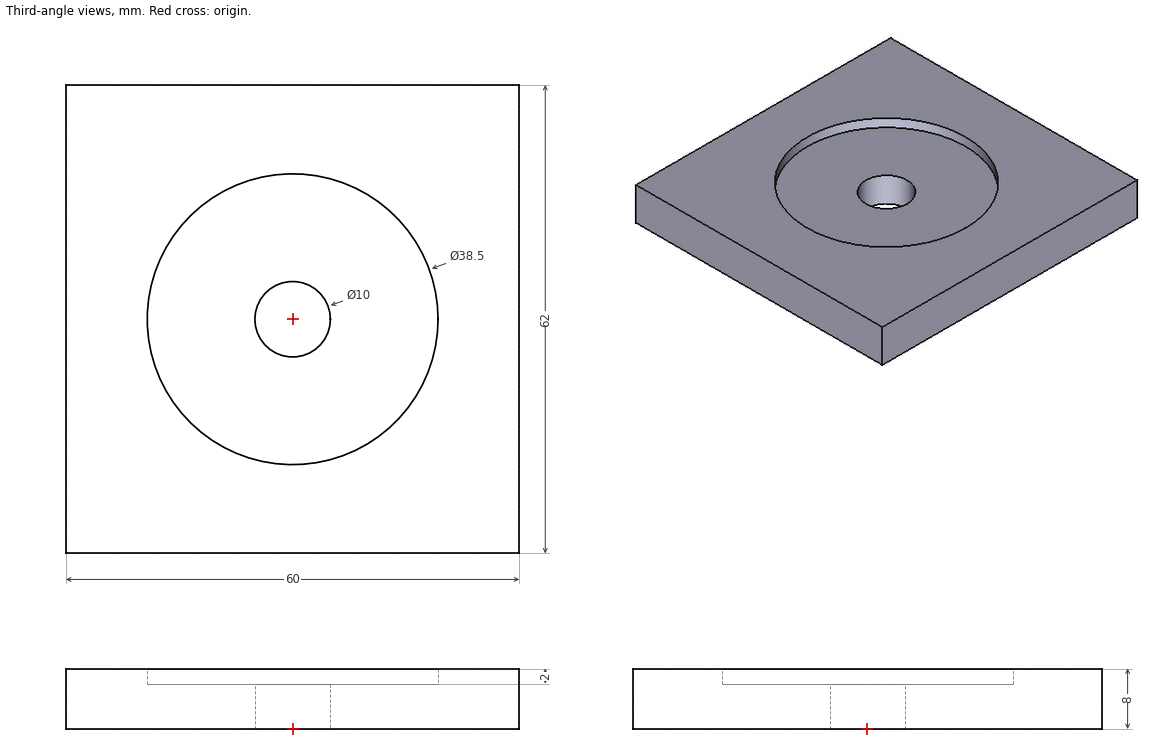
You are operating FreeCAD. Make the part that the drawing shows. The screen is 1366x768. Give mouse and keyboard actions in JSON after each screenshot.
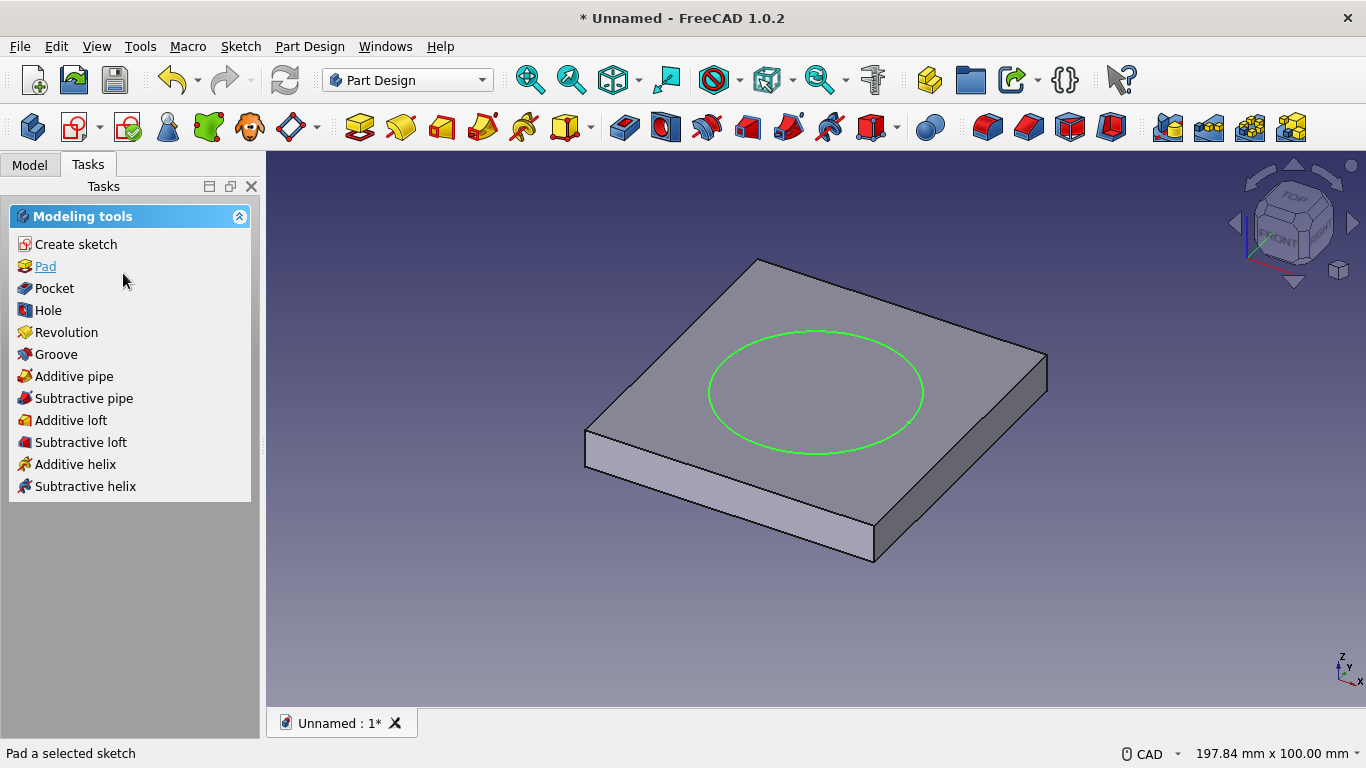
{"action": "left_click", "coordinate": [625, 128]}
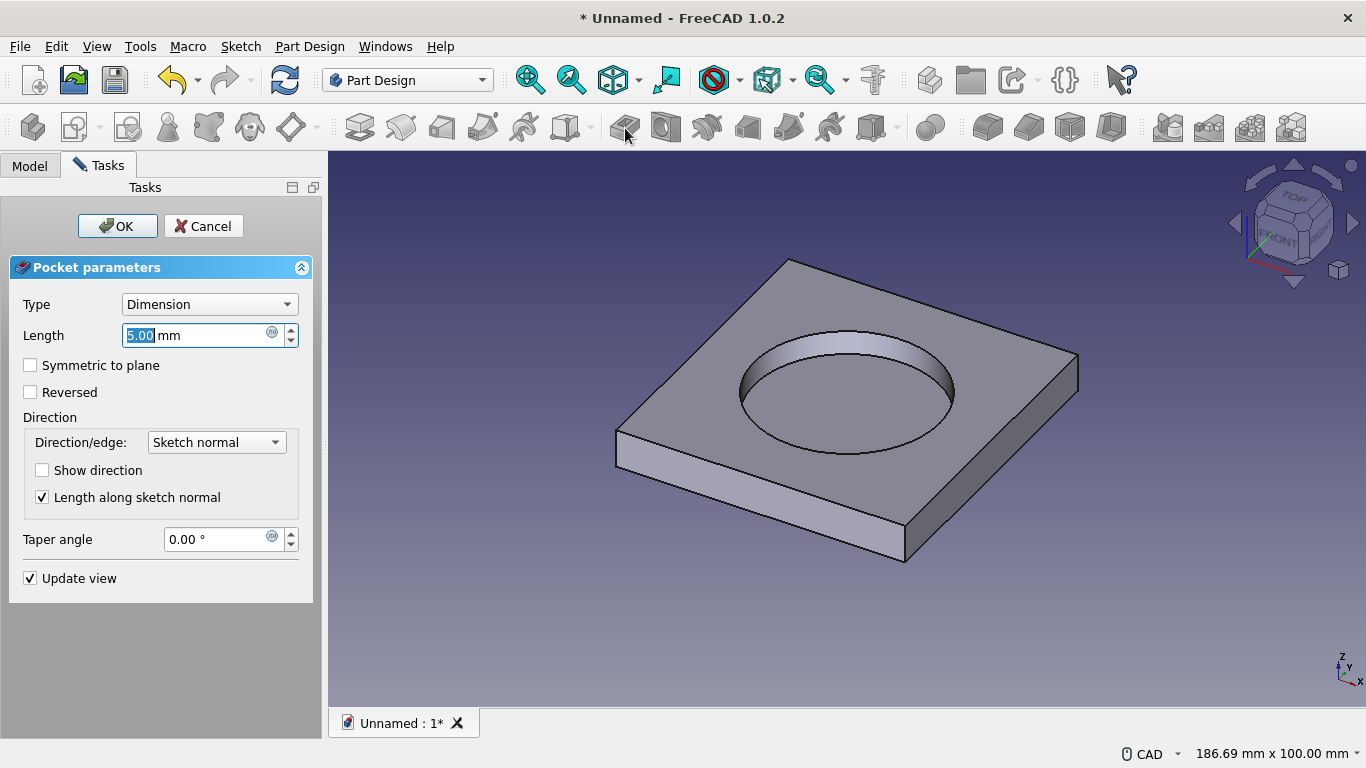
{"action": "type", "text": "2"}
{"action": "key", "text": "Tab"}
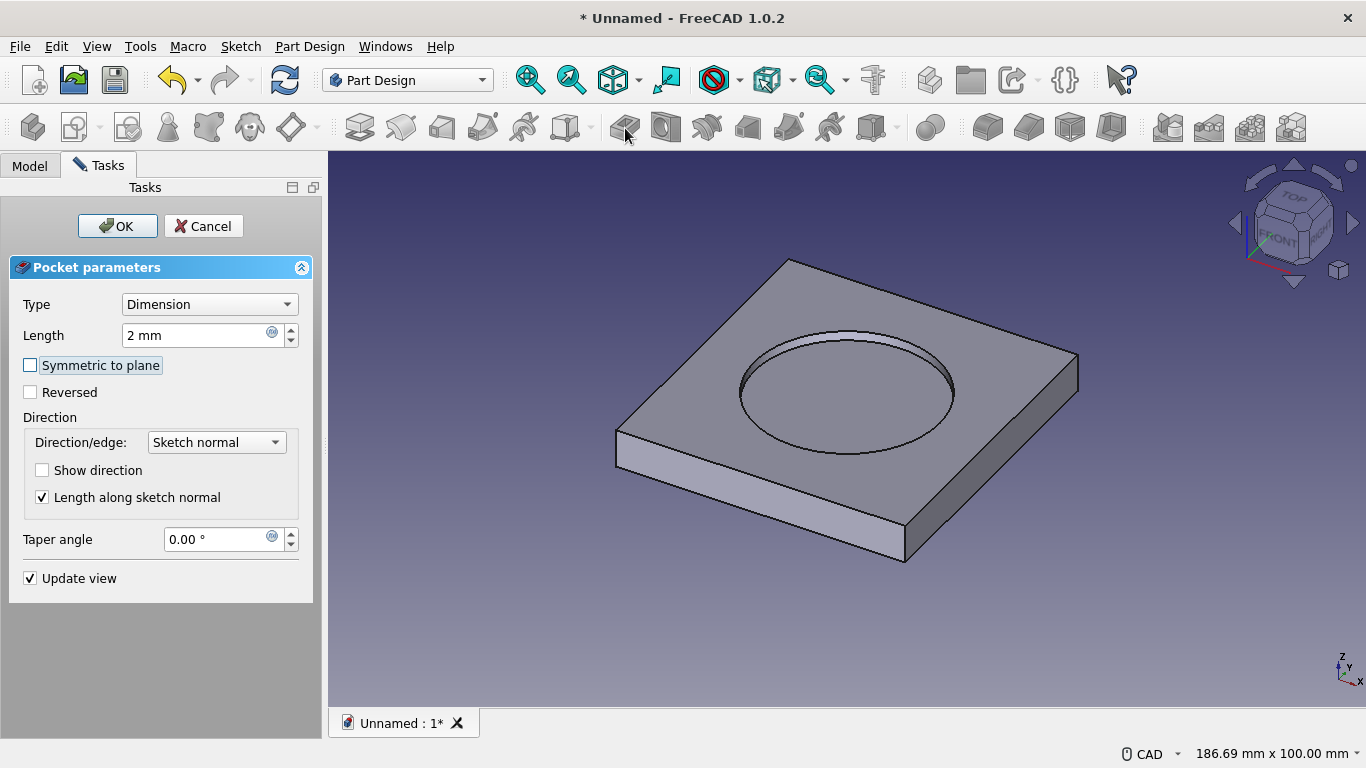
{"action": "left_click", "coordinate": [118, 226]}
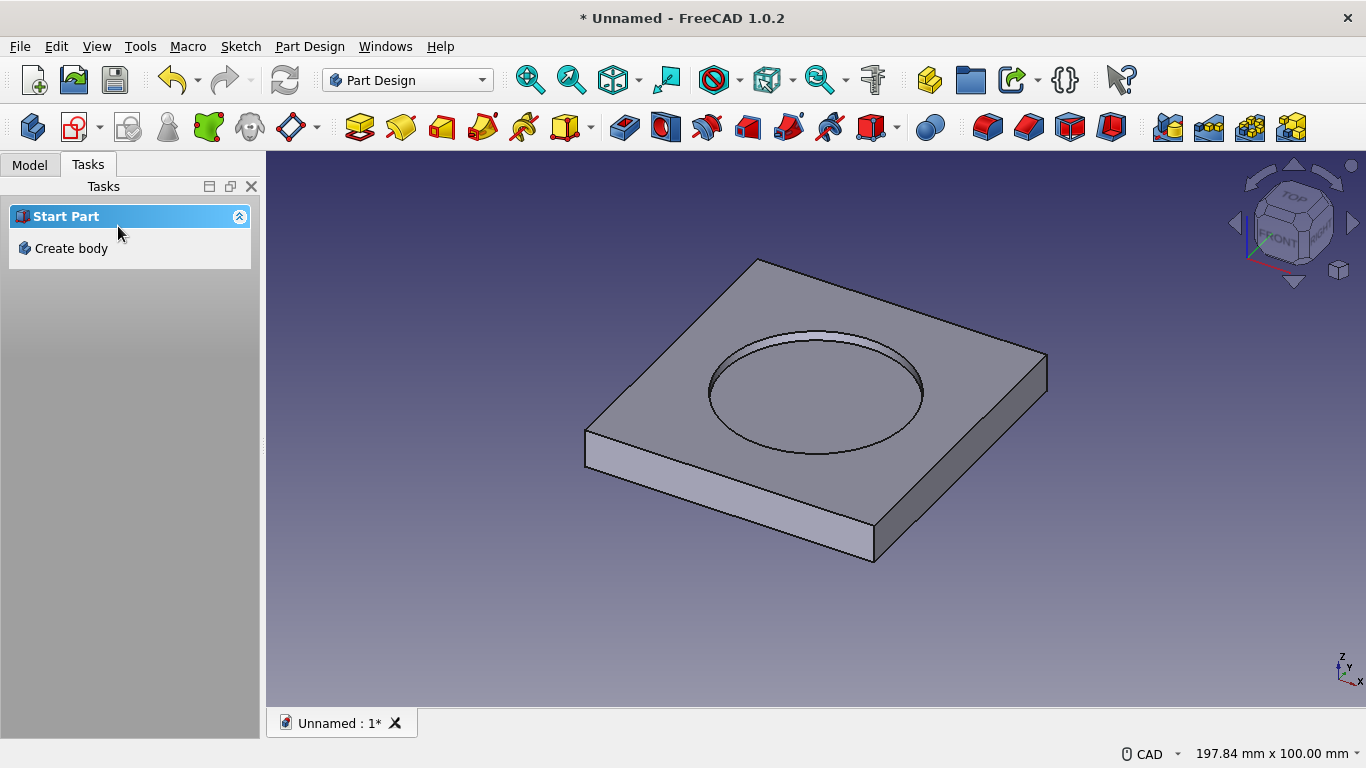
{"action": "left_click", "coordinate": [816, 401]}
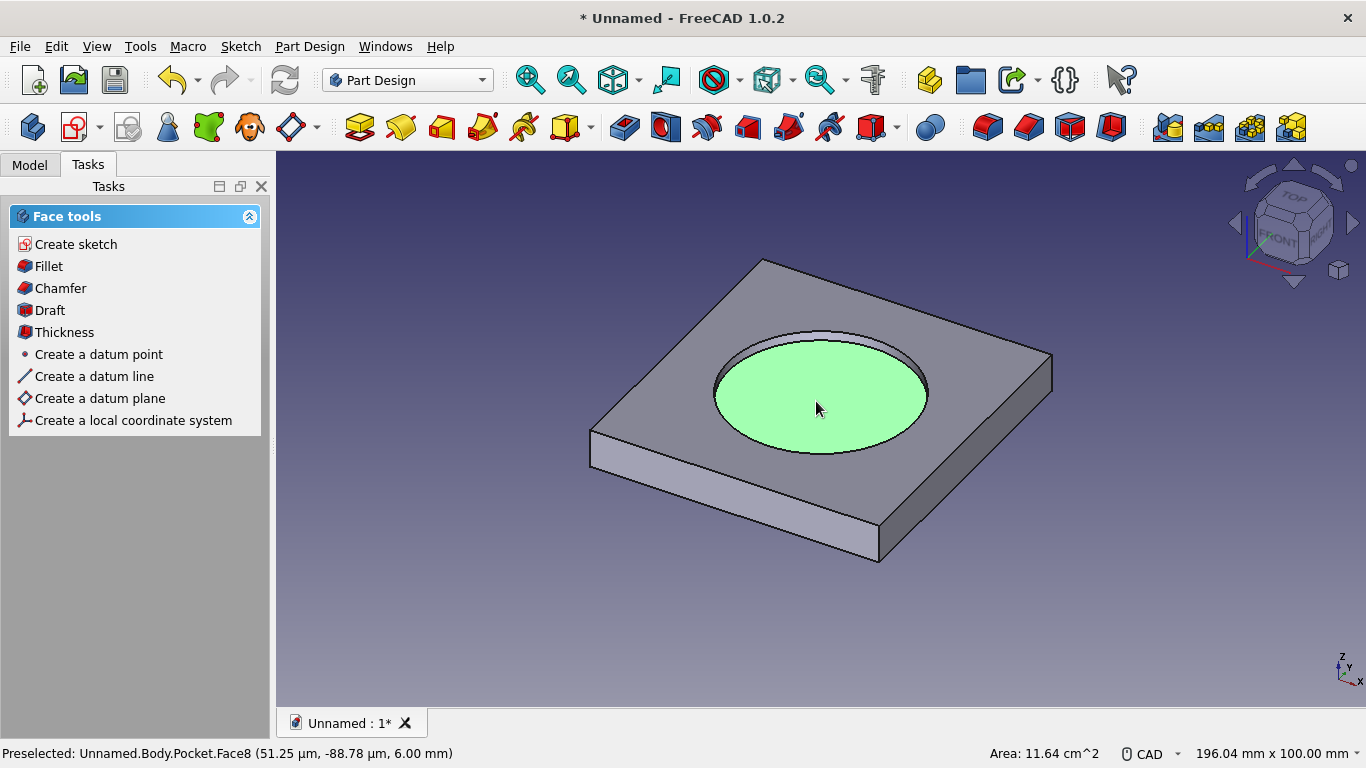
{"action": "left_click", "coordinate": [74, 128]}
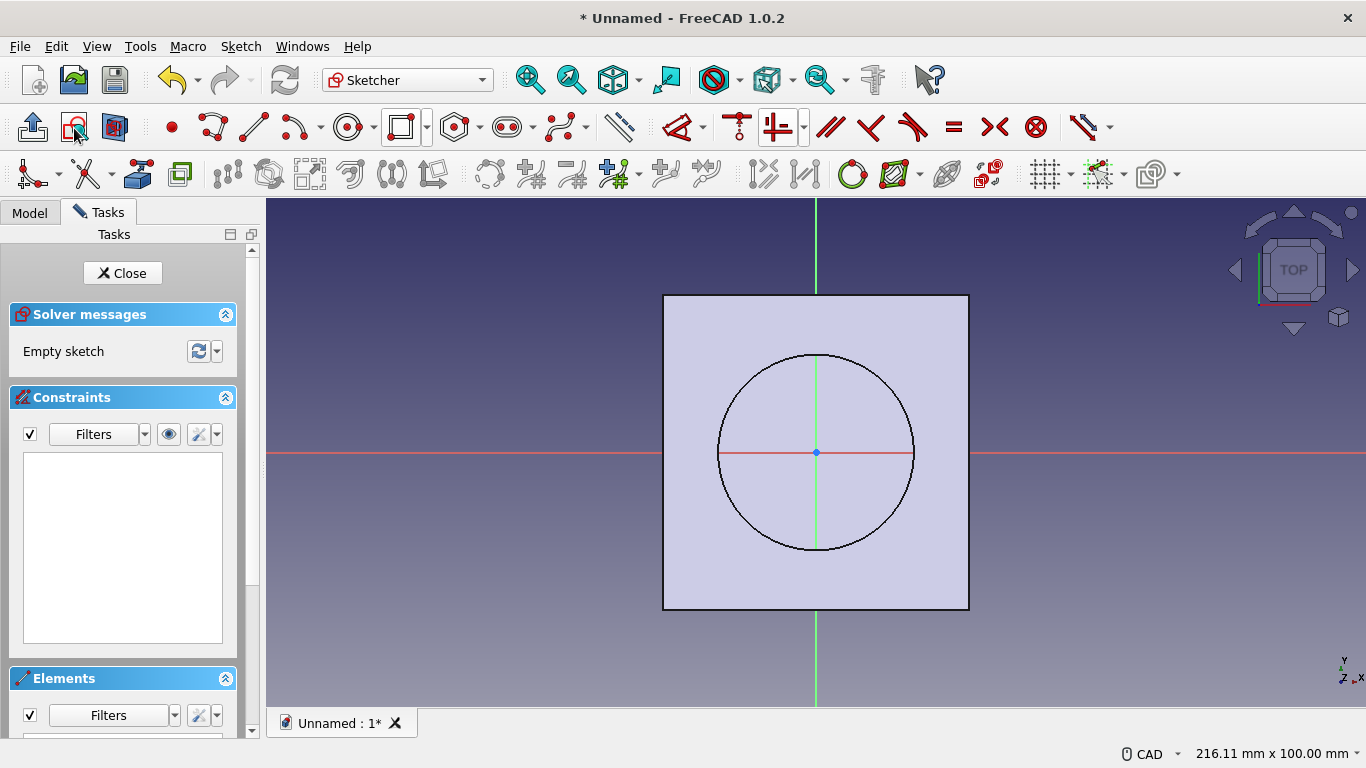
{"action": "left_click", "coordinate": [115, 128]}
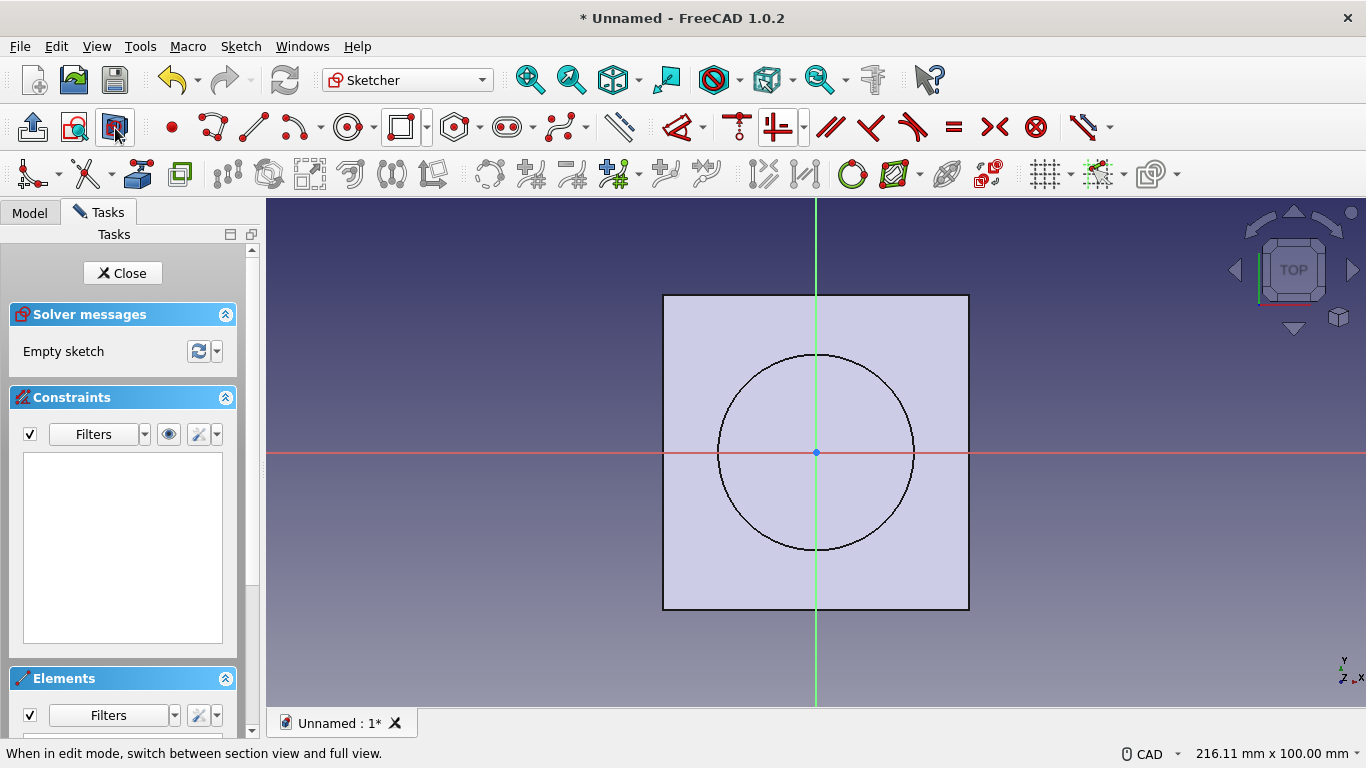
{"action": "scroll", "coordinate": [830, 452], "scroll_direction": "up", "scroll_amount": 9}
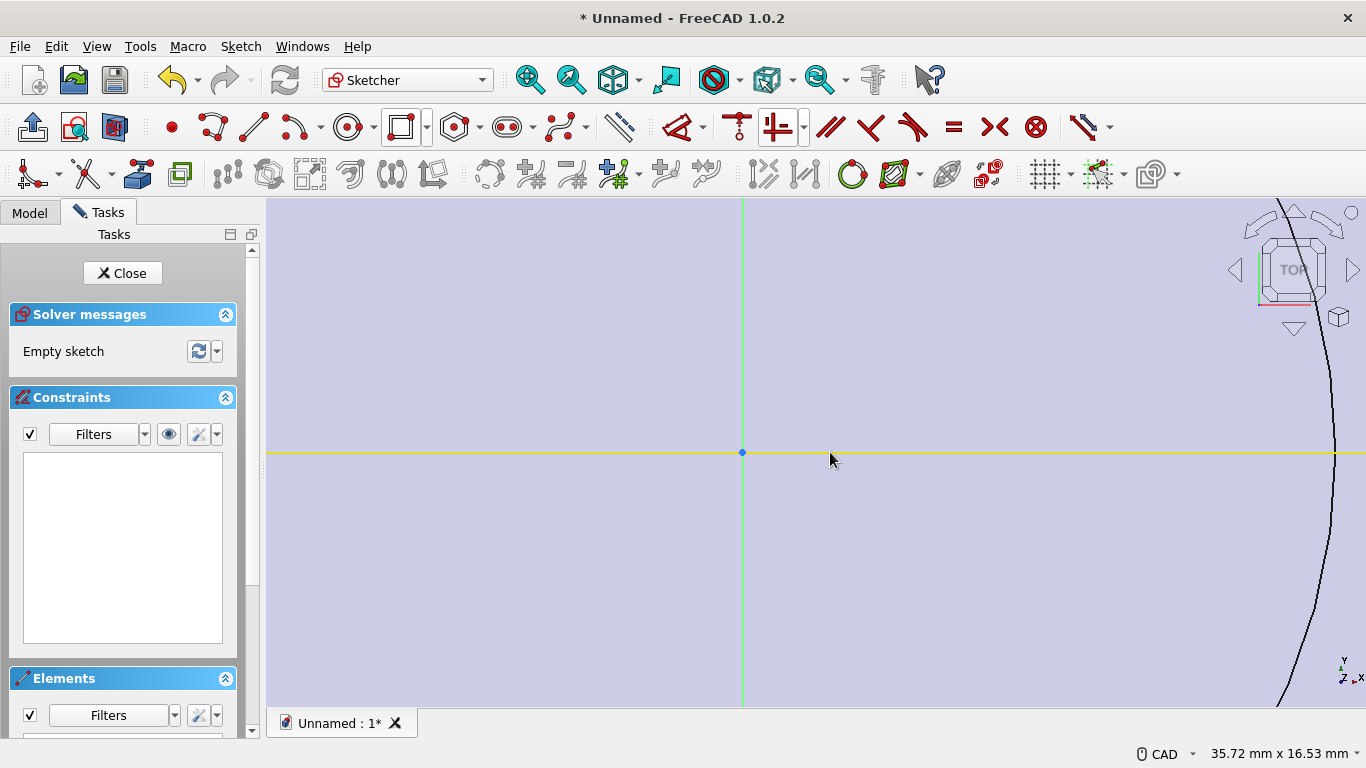
{"action": "left_click", "coordinate": [348, 128]}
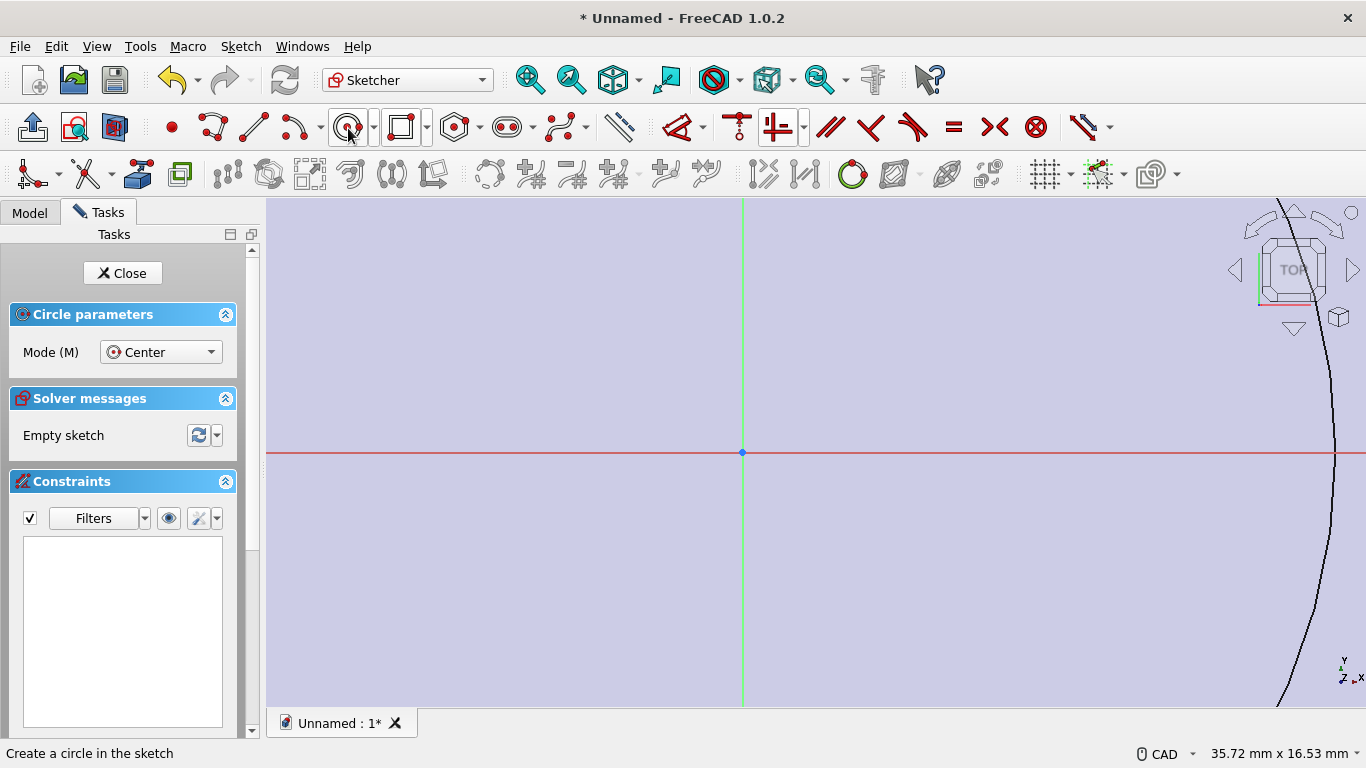
{"action": "left_click", "coordinate": [743, 452]}
{"action": "mouse_move", "coordinate": [852, 344]}